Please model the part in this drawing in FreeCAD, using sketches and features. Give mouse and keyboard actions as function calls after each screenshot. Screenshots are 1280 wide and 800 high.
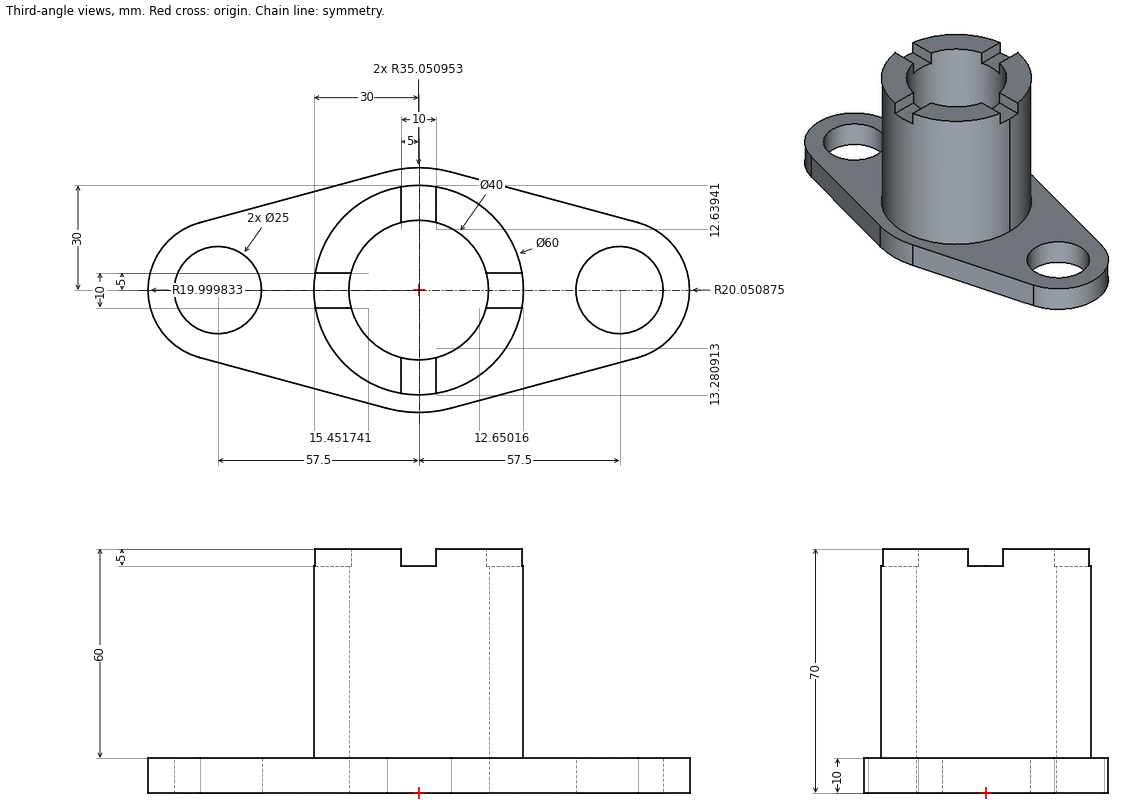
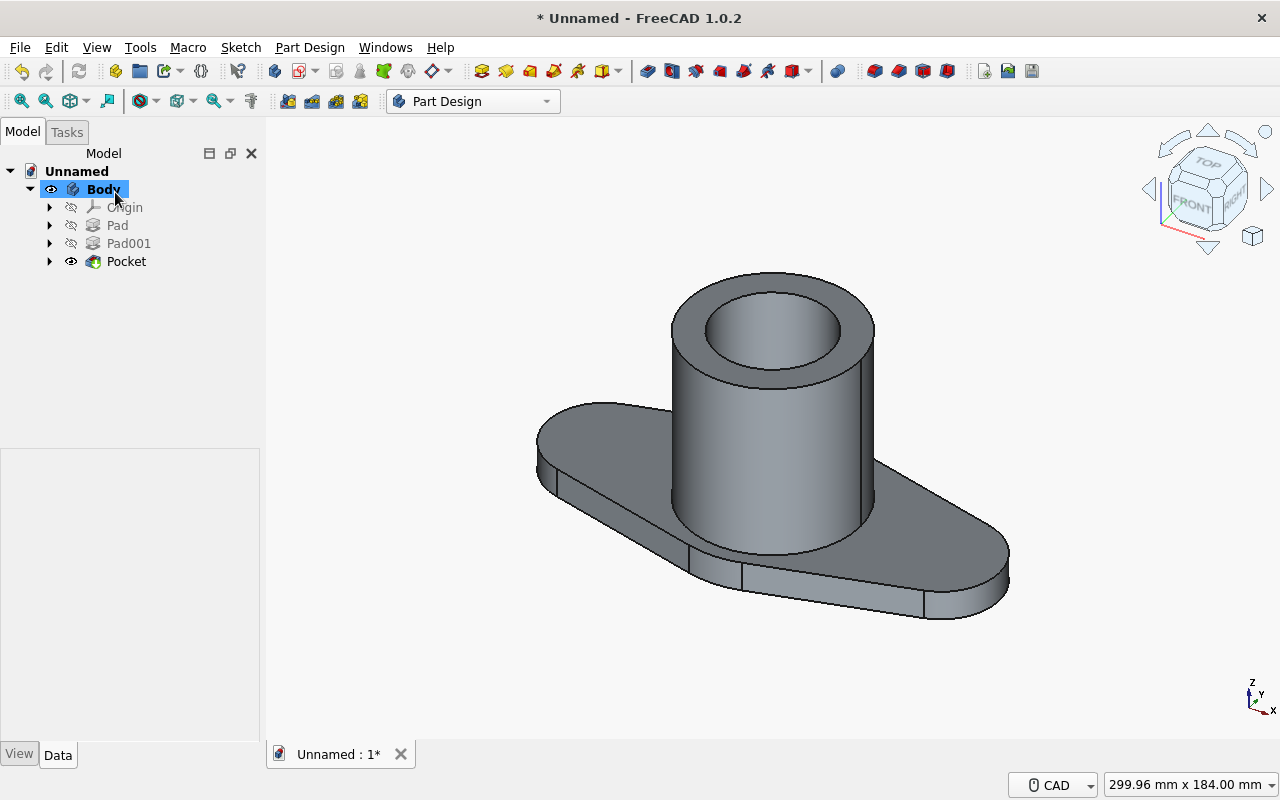
click(848, 355)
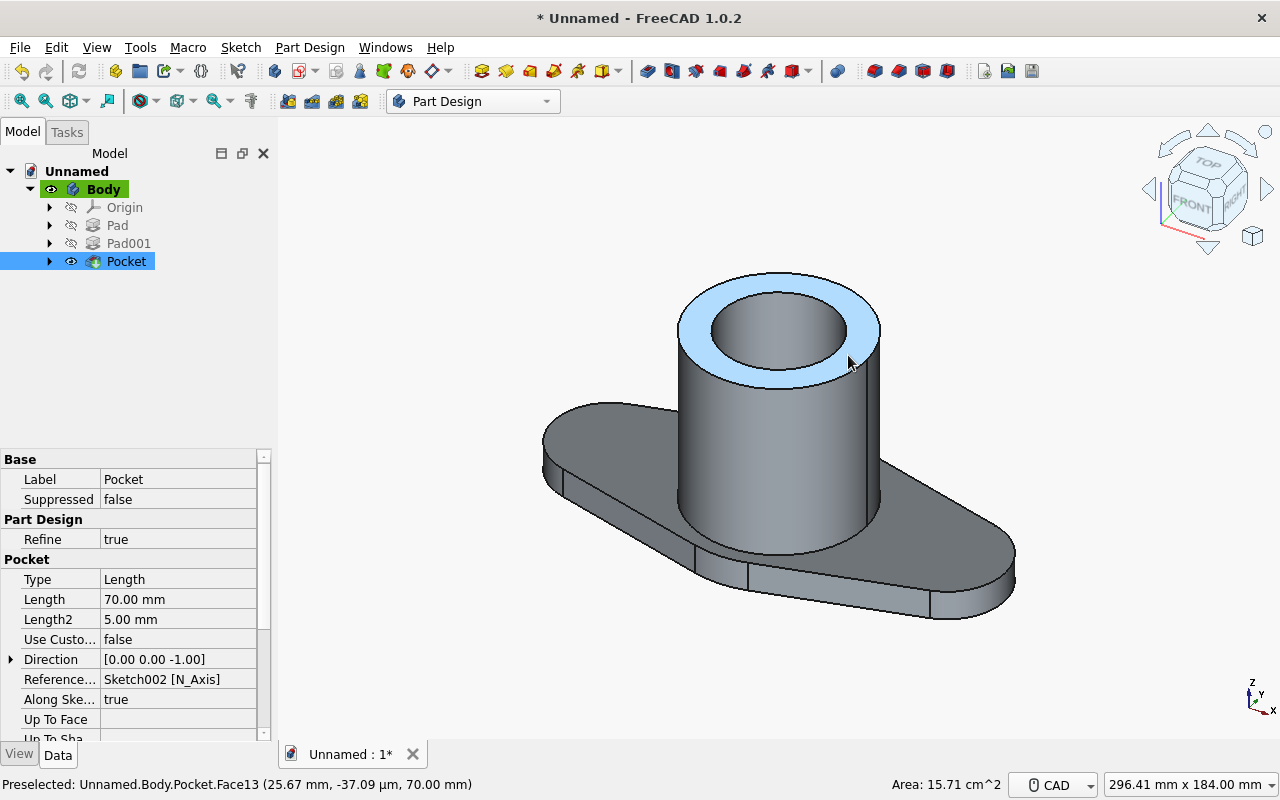
click(300, 72)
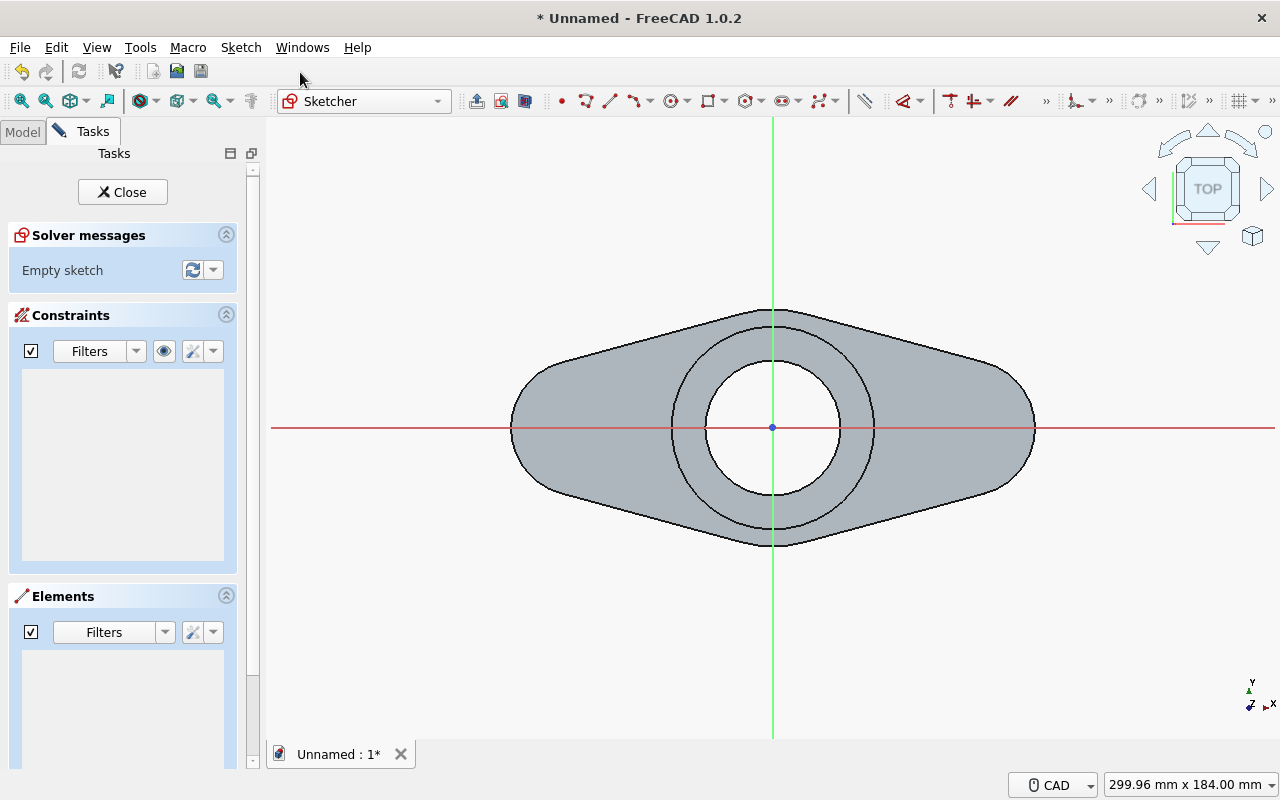
scroll(856, 428, up, 3)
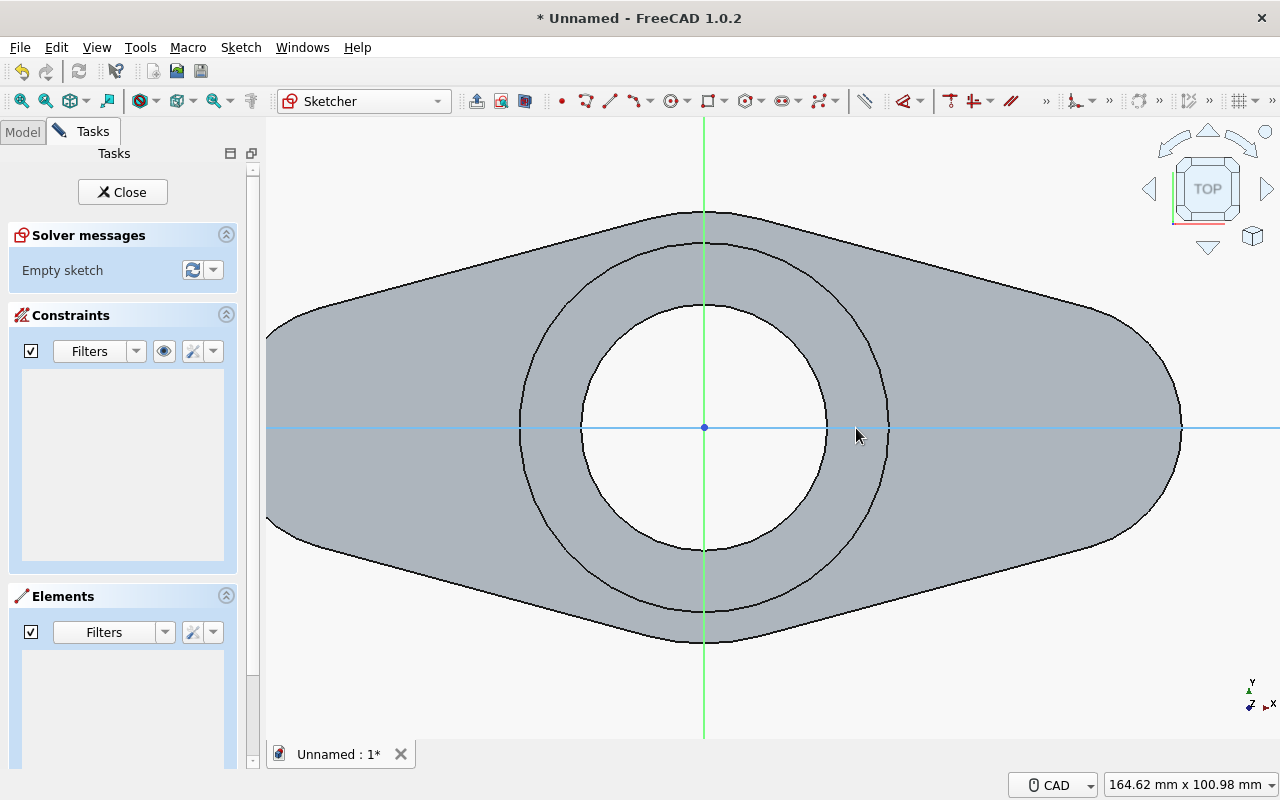
click(708, 102)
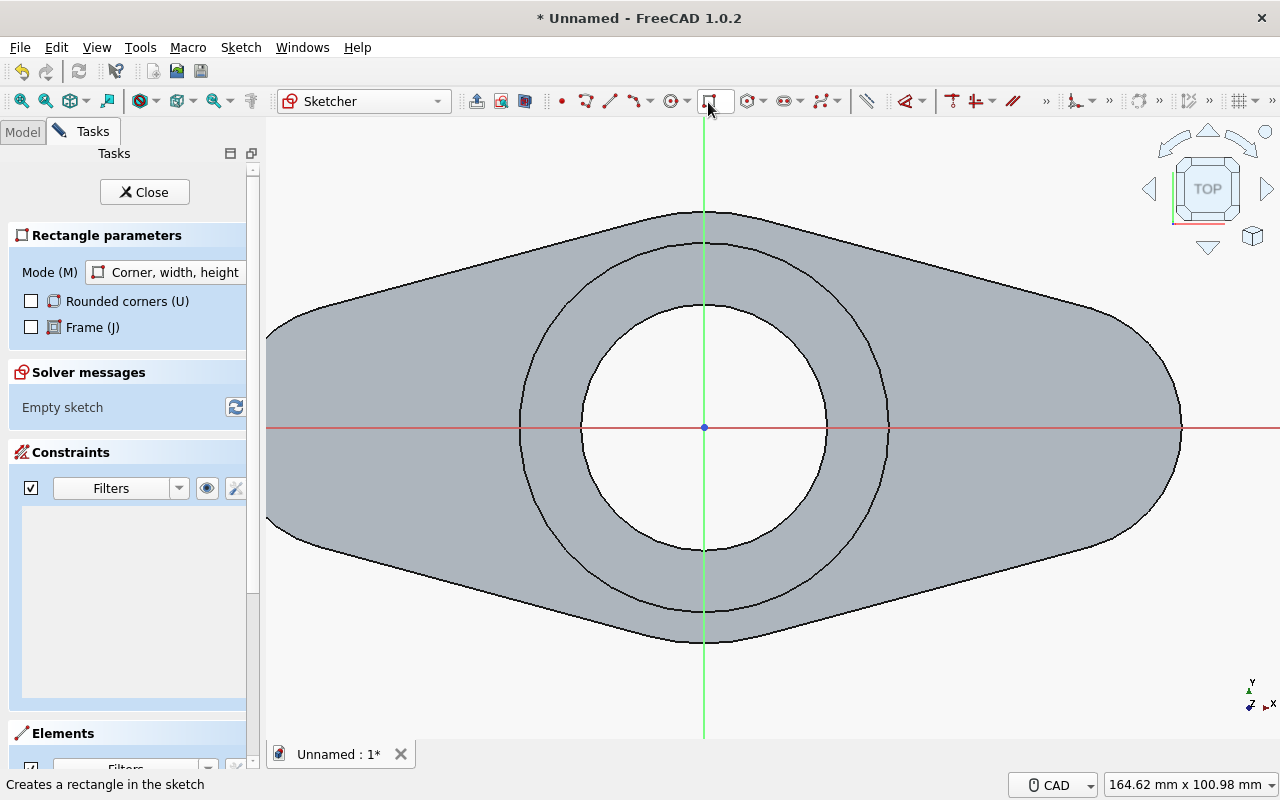
click(673, 243)
move(735, 321)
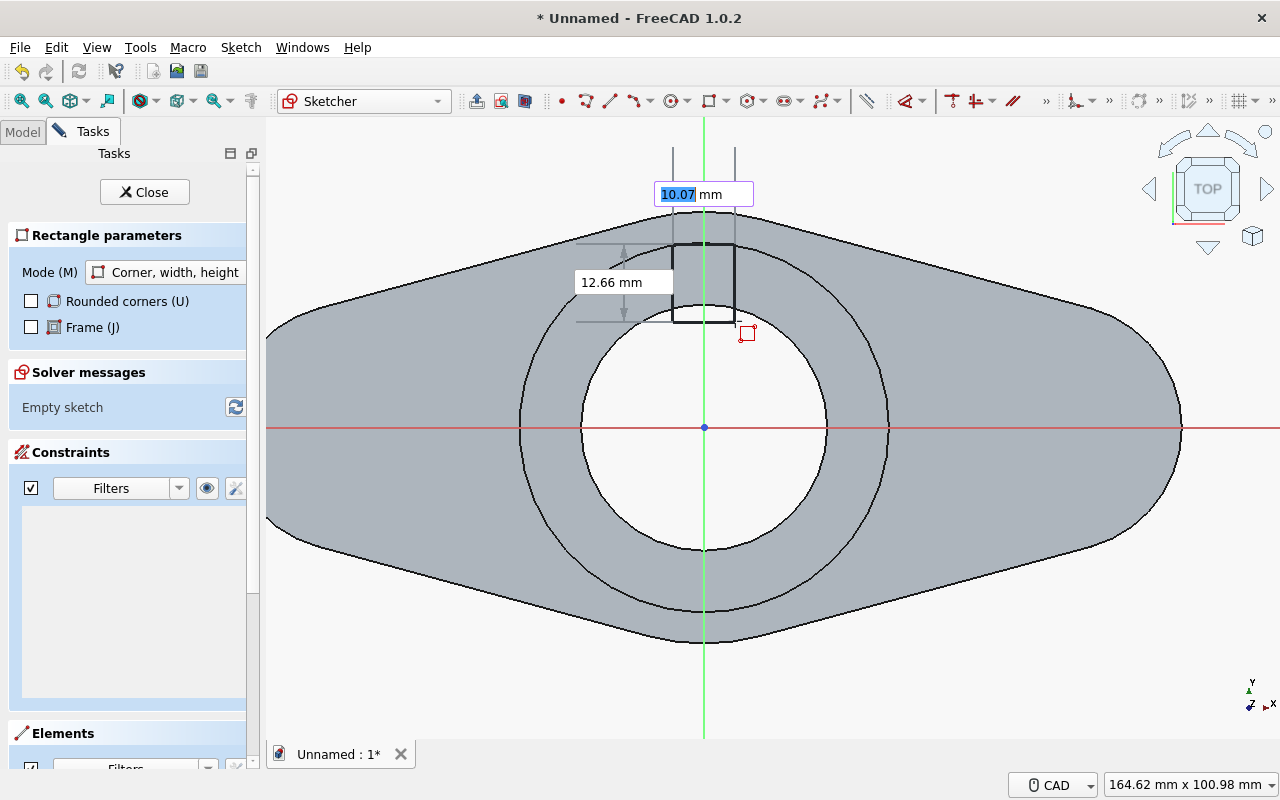
text(10)
key(Tab)
text(12.63941)
key(Return)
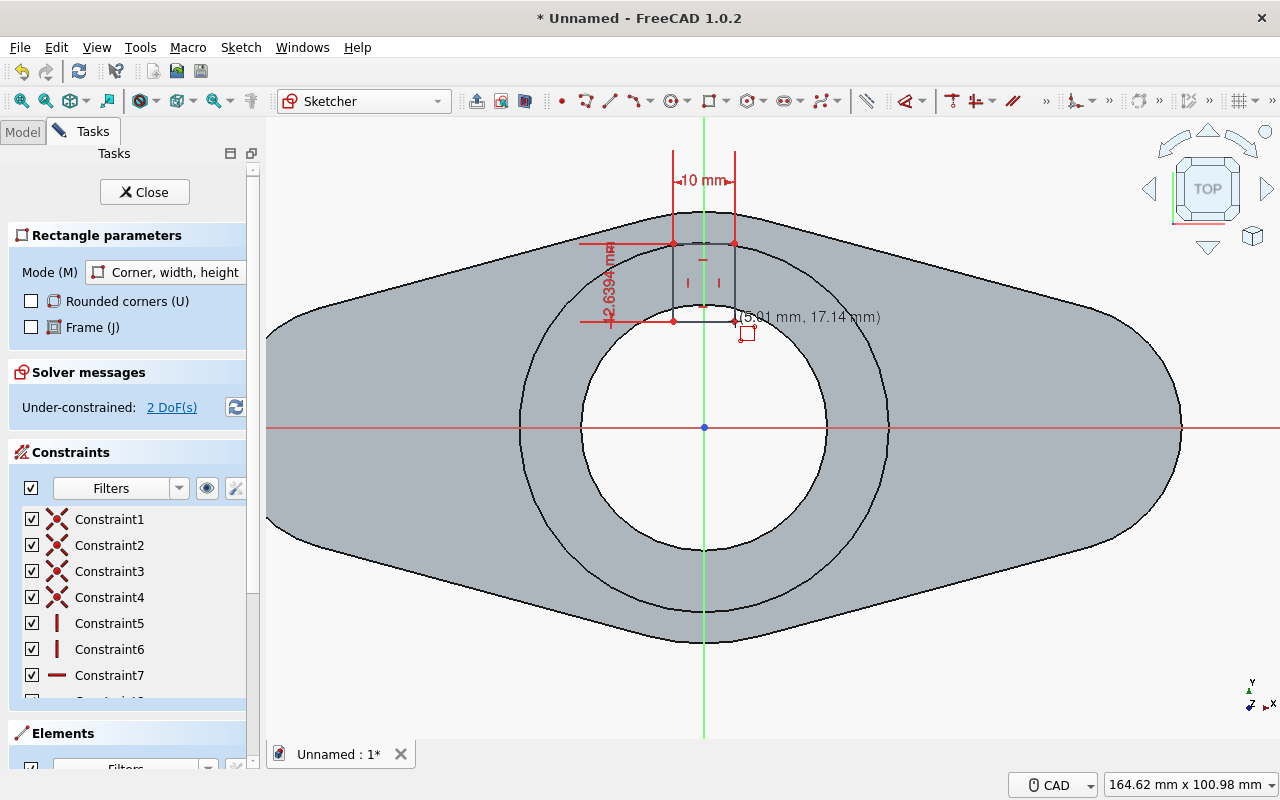
click(673, 531)
move(735, 612)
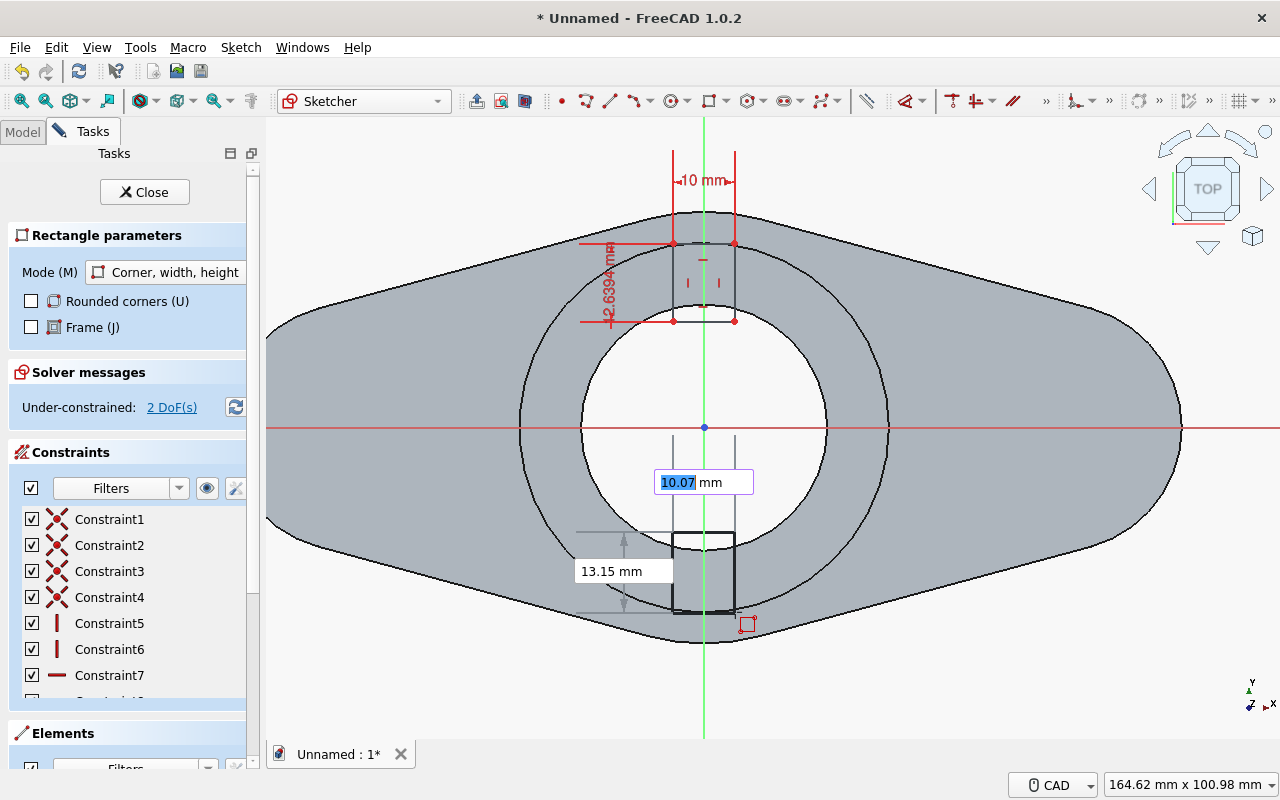
text(10)
key(Tab)
text(13.280913)
key(Return)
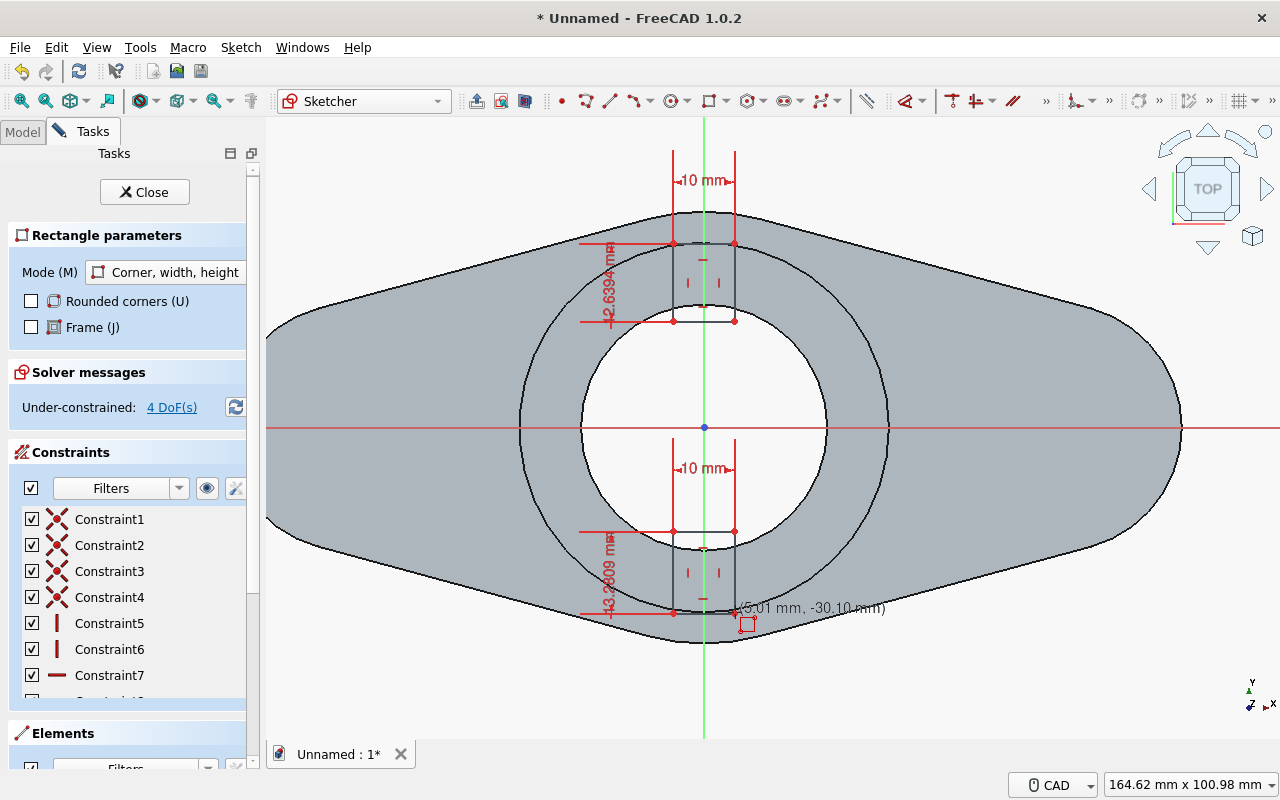
click(519, 397)
move(615, 458)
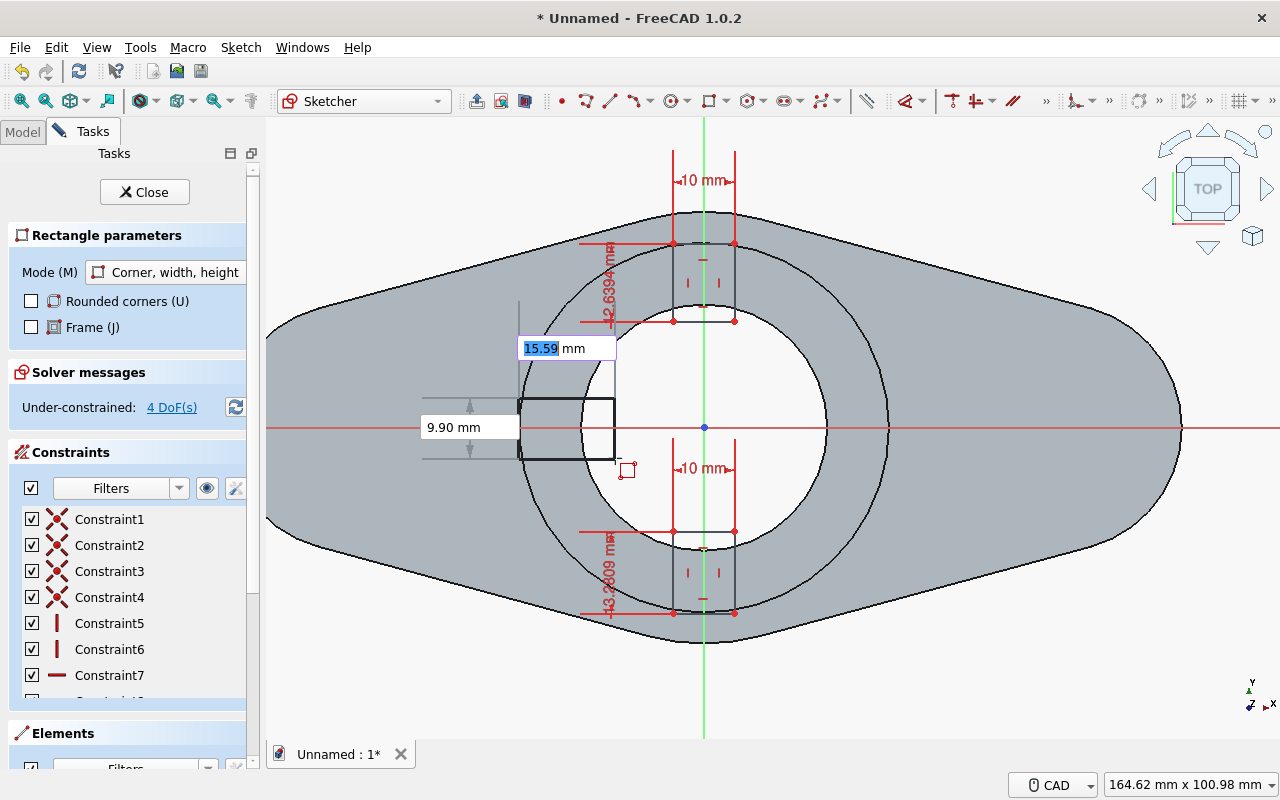
text(15.451741)
key(Tab)
text(10)
key(Return)